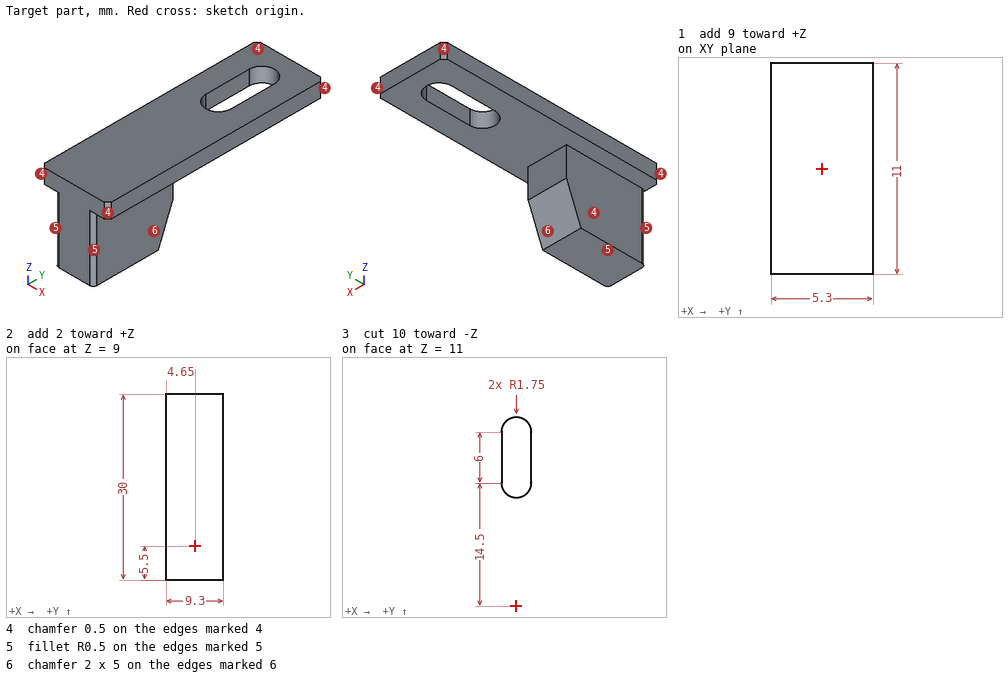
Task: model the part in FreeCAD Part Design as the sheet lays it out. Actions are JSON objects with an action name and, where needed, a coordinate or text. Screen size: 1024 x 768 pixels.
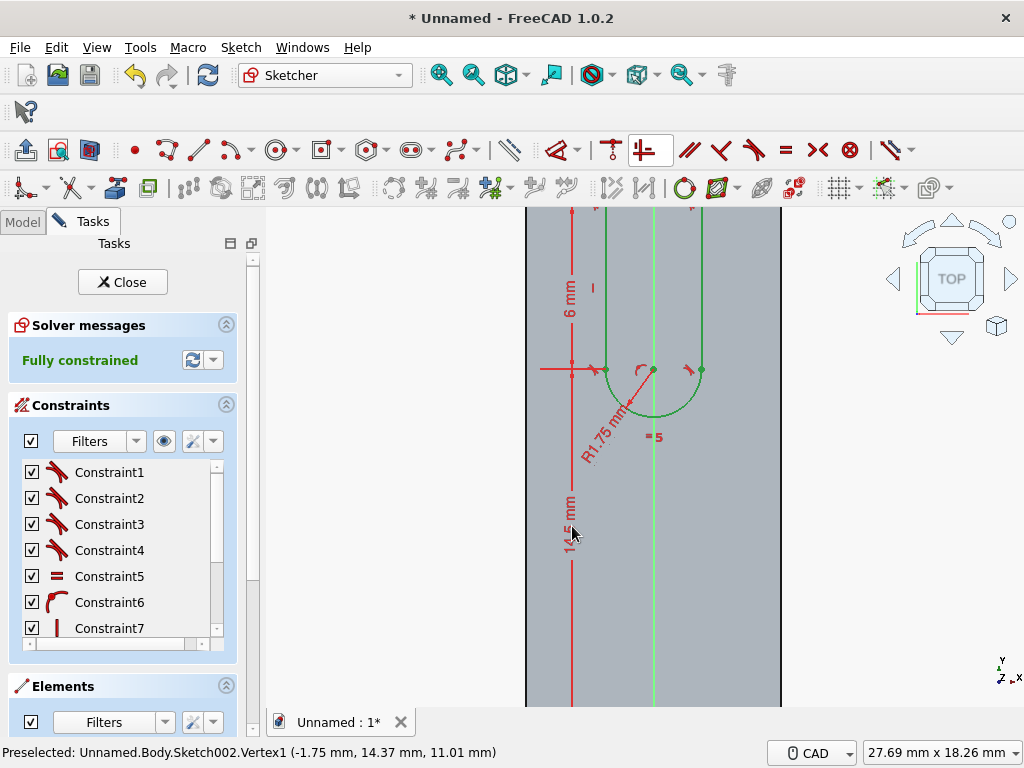
{"action": "left_click", "coordinate": [123, 282]}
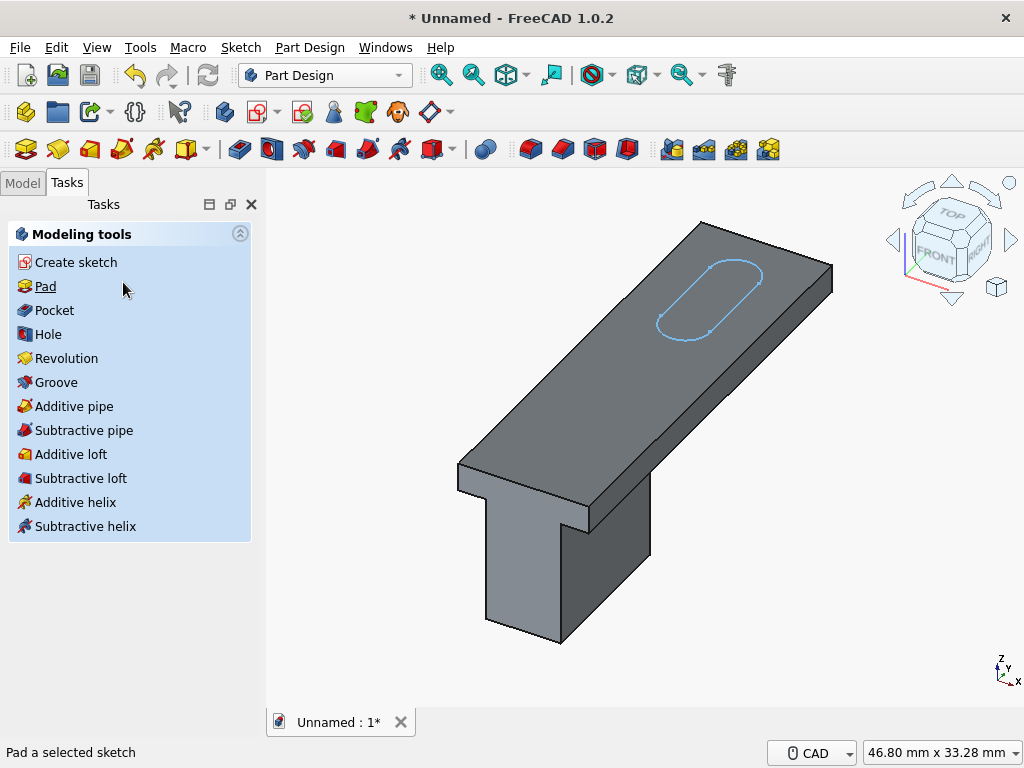
{"action": "left_click", "coordinate": [240, 150]}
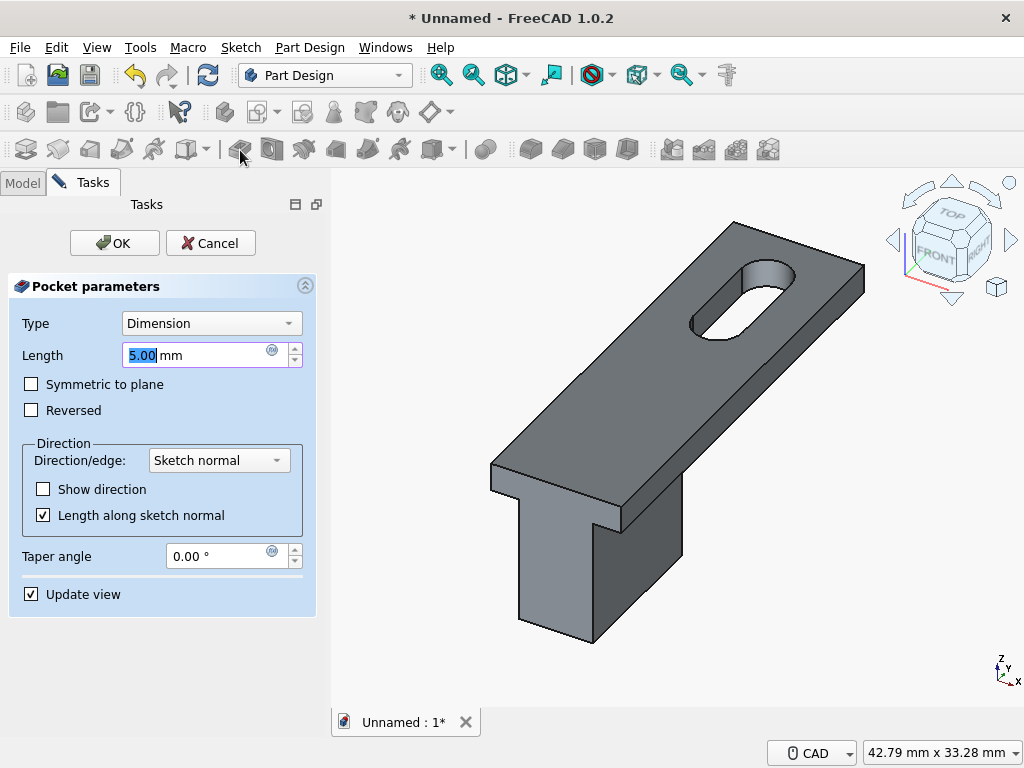
{"action": "type", "text": "10"}
{"action": "key", "text": "Tab"}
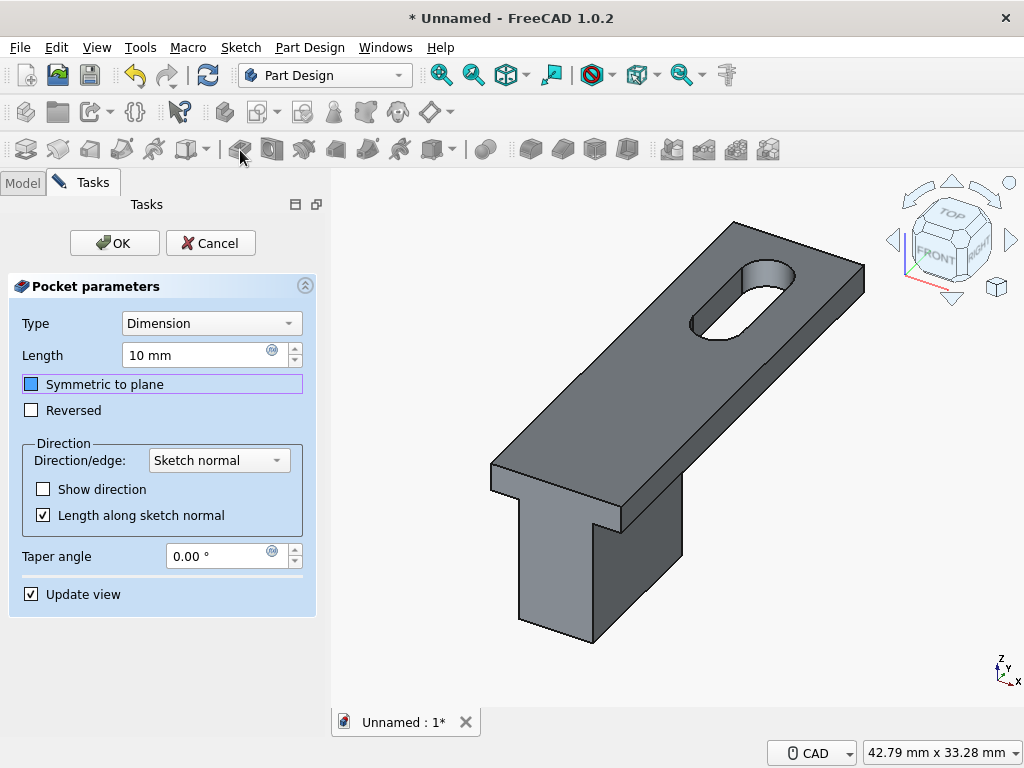
{"action": "left_click", "coordinate": [115, 243]}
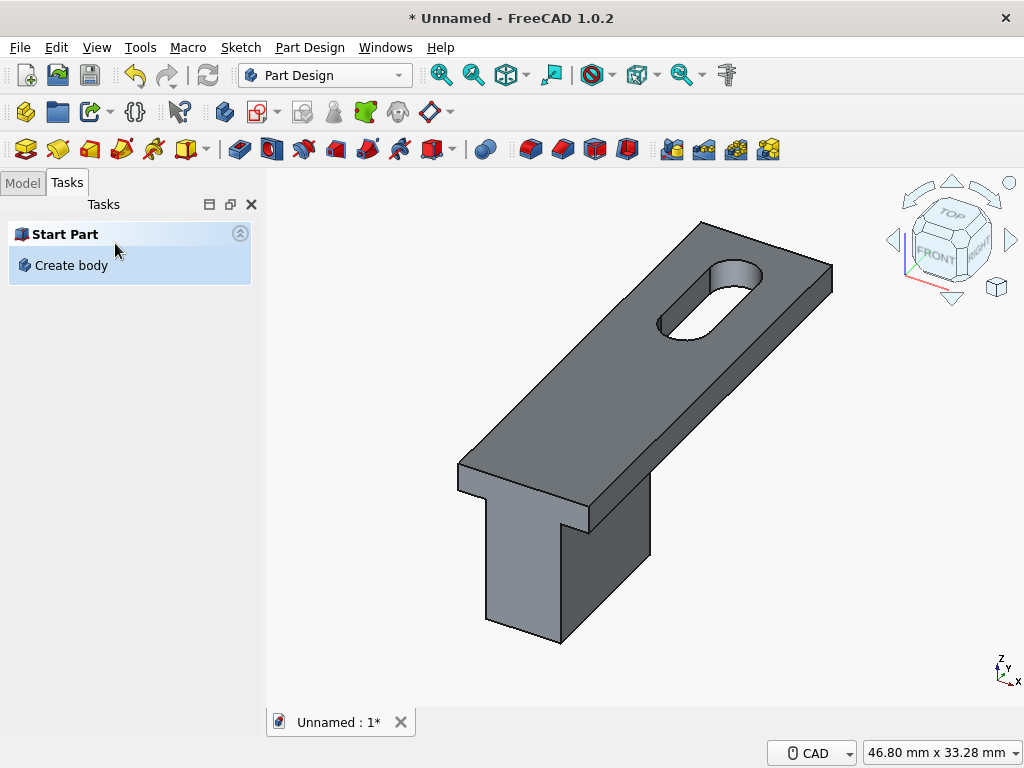
{"action": "left_click", "coordinate": [589, 519]}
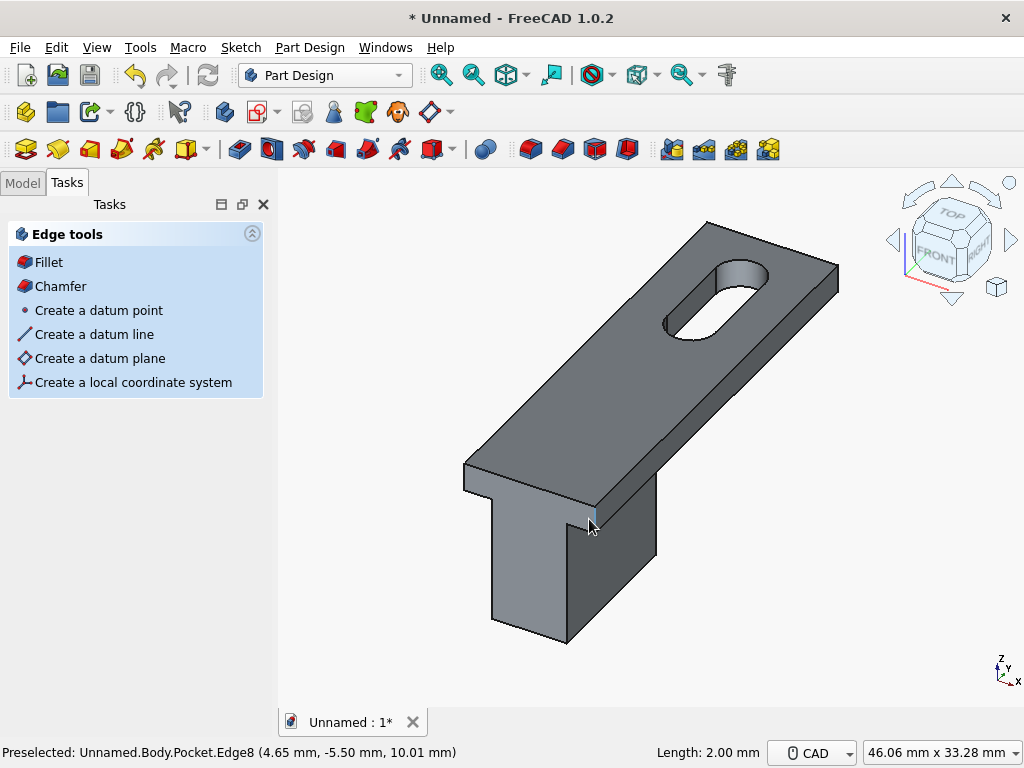
{"action": "key", "text": "0"}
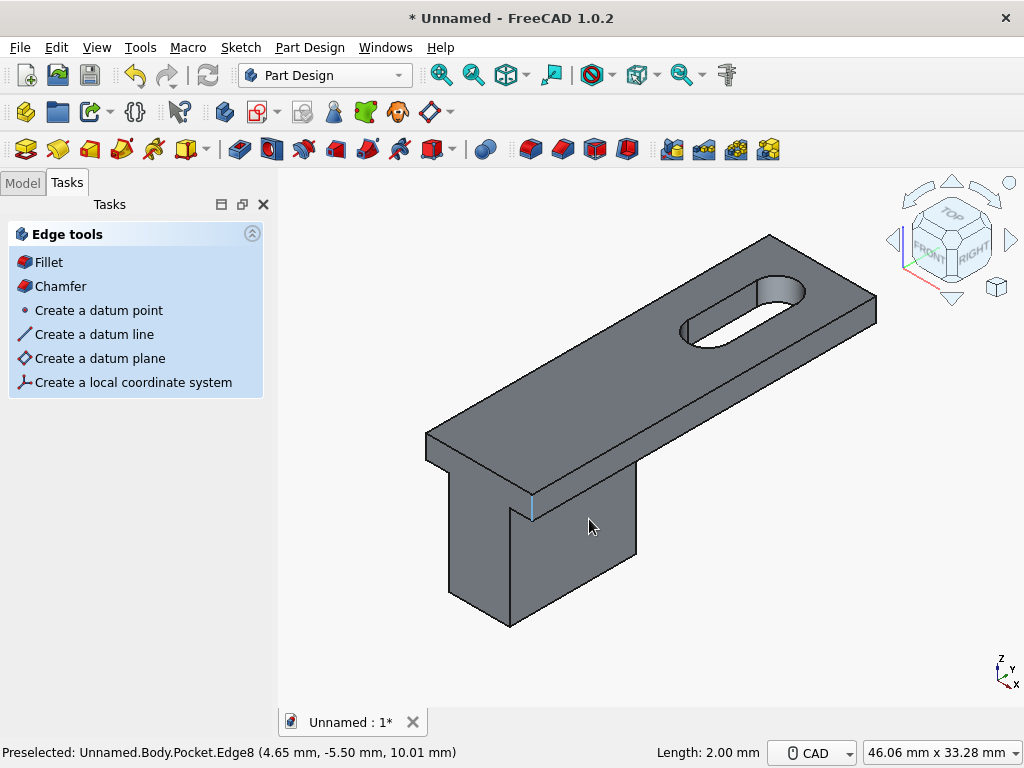
{"action": "key", "text": "2"}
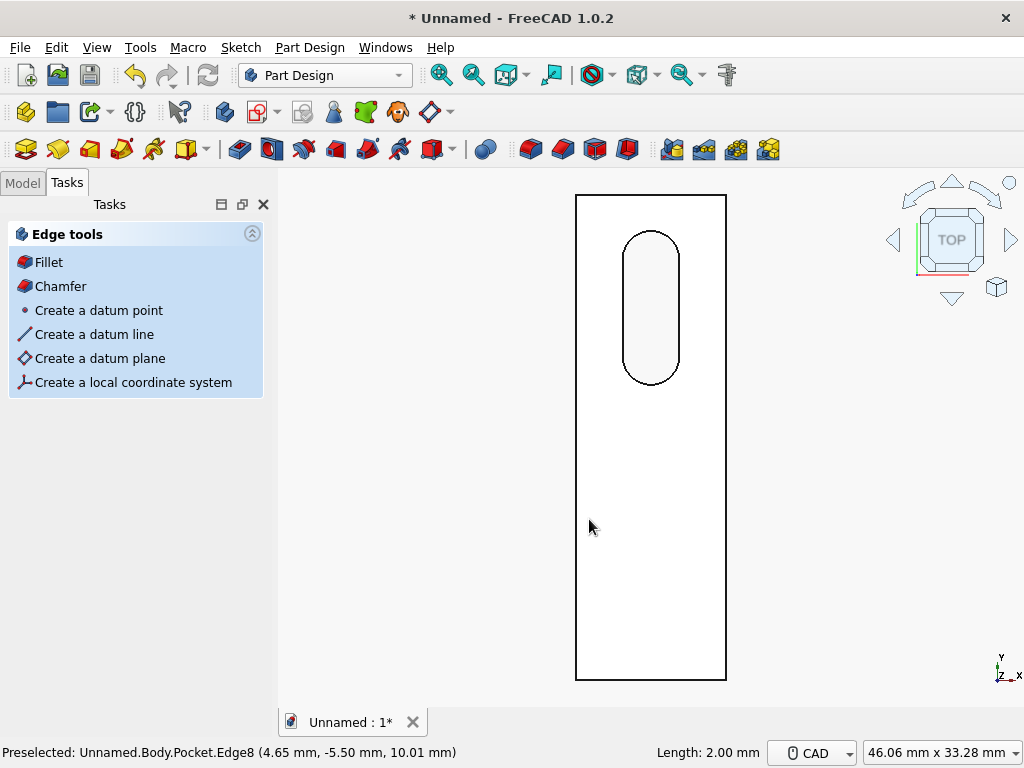
{"action": "key", "text": "1"}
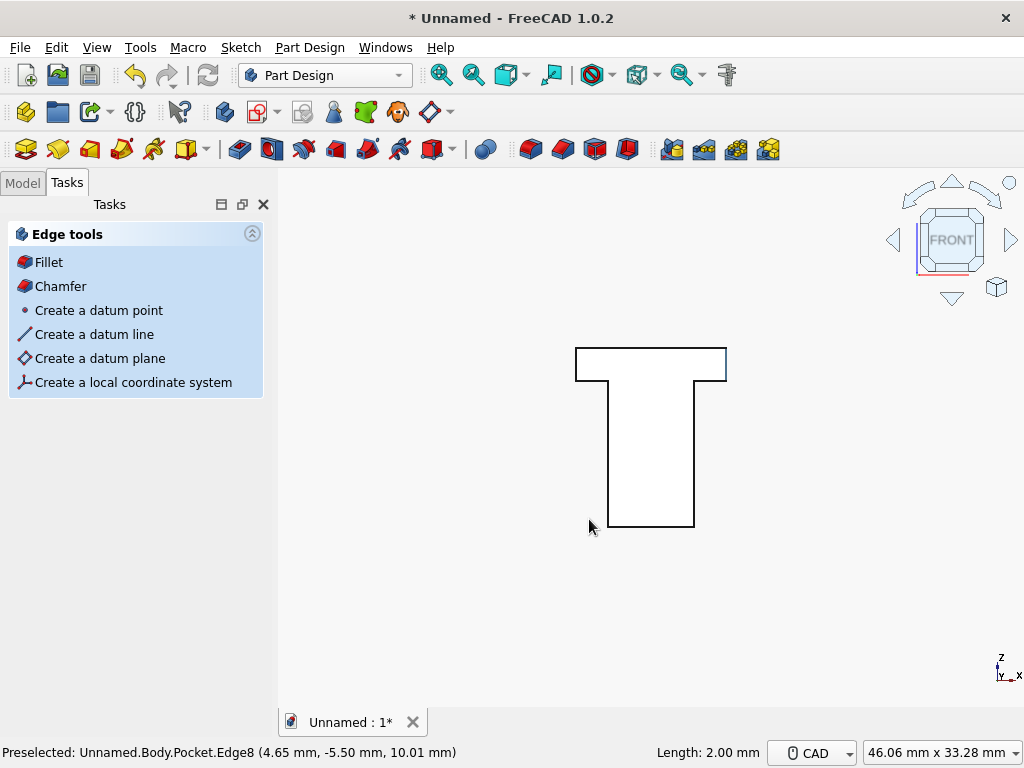
{"action": "left_click", "coordinate": [442, 76]}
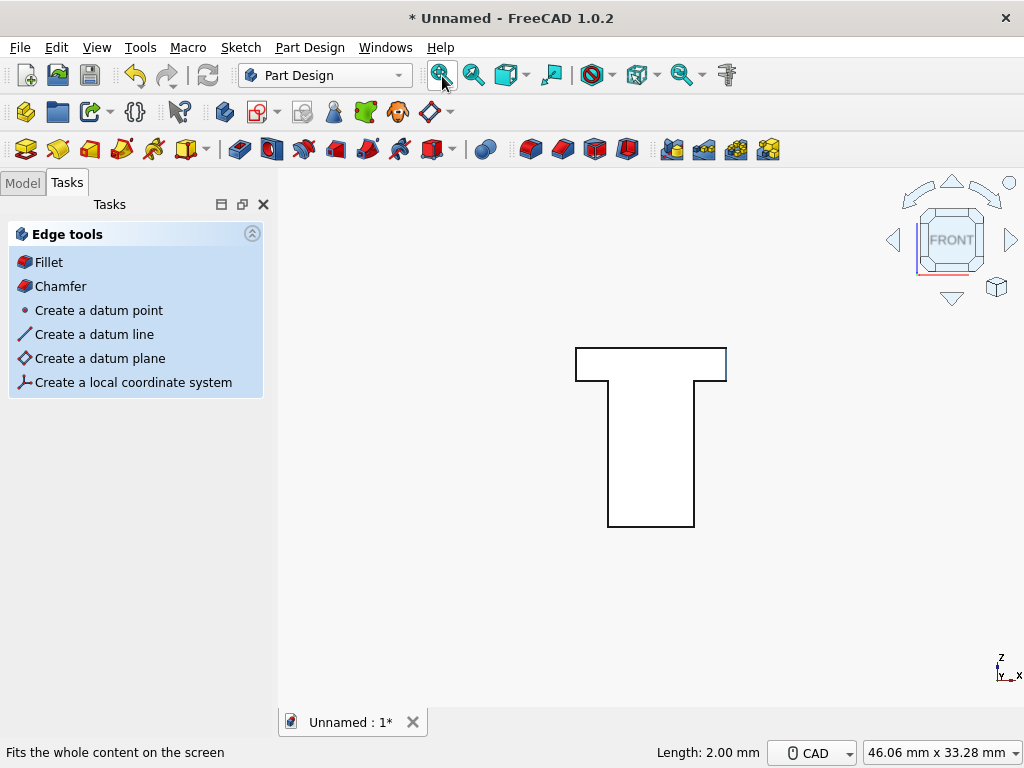
{"action": "left_click", "coordinate": [576, 364], "text": "ctrl"}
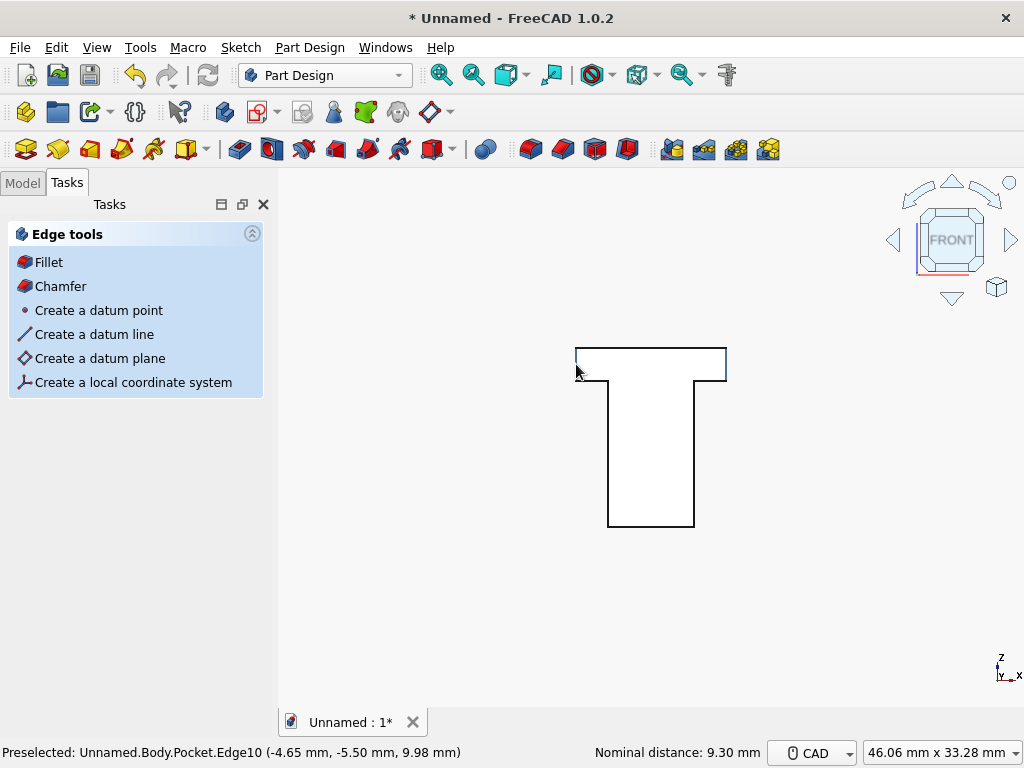
{"action": "key", "text": "3"}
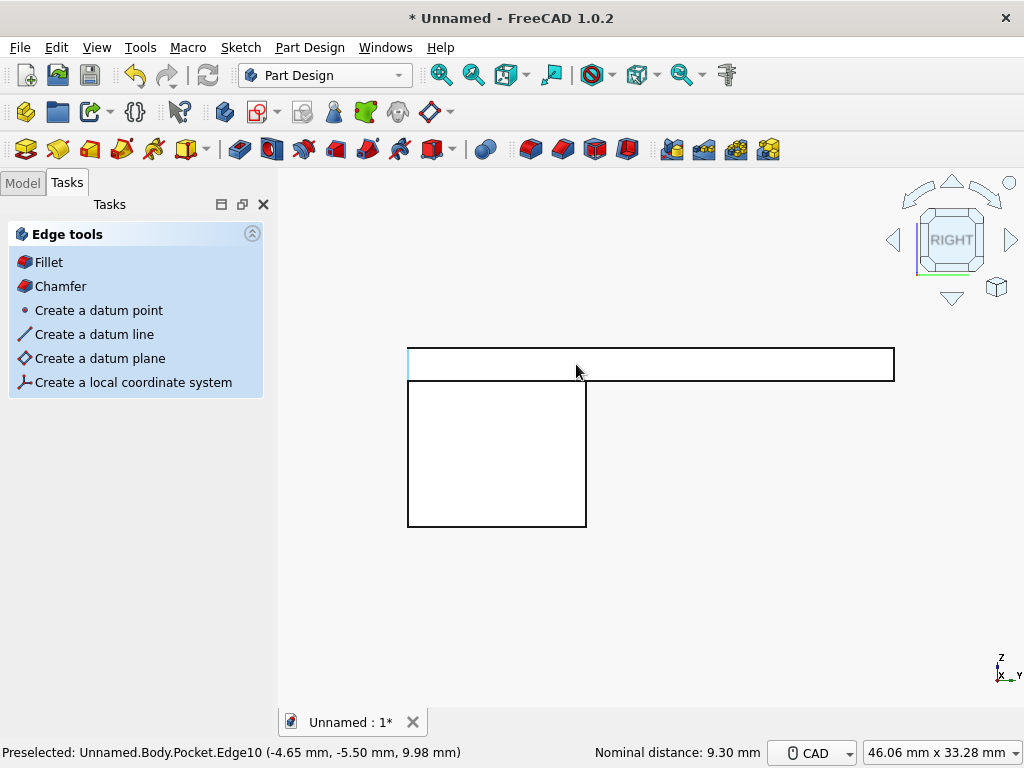
{"action": "left_click", "coordinate": [894, 364], "text": "ctrl"}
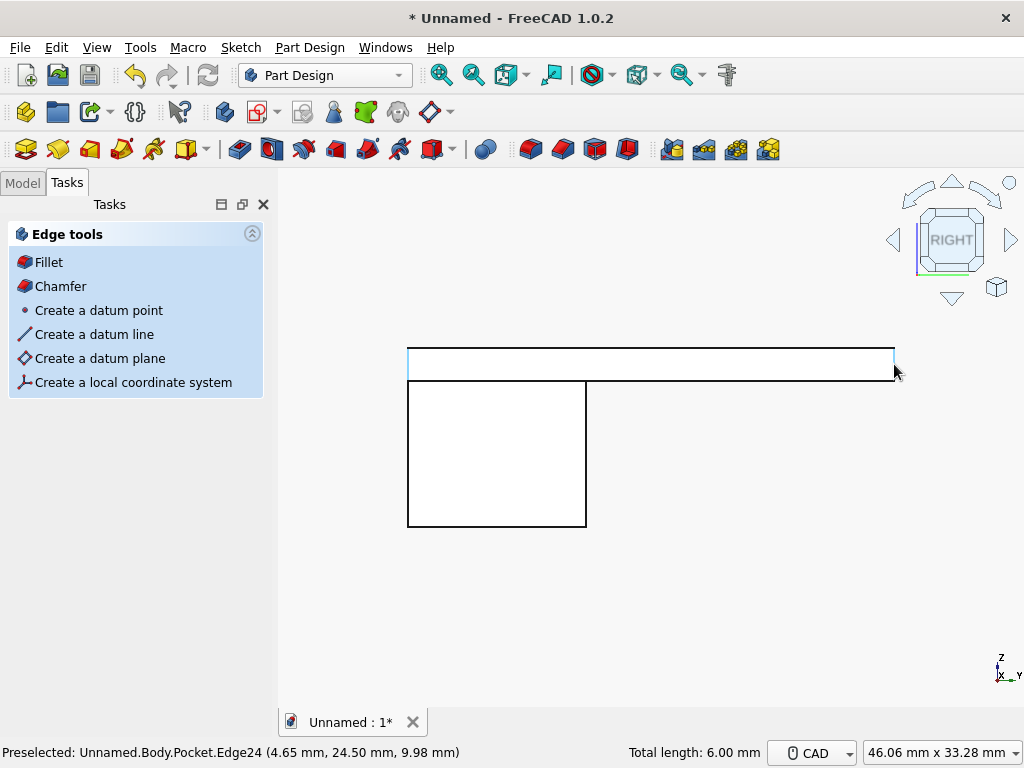
{"action": "key", "text": "5"}